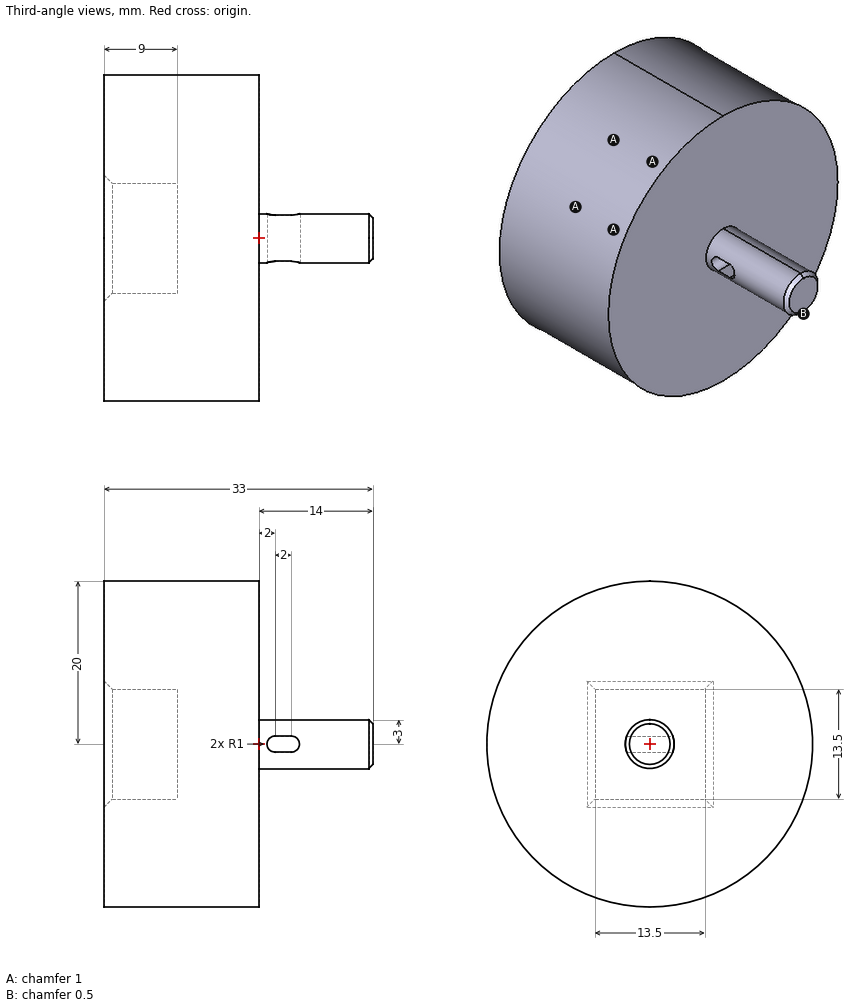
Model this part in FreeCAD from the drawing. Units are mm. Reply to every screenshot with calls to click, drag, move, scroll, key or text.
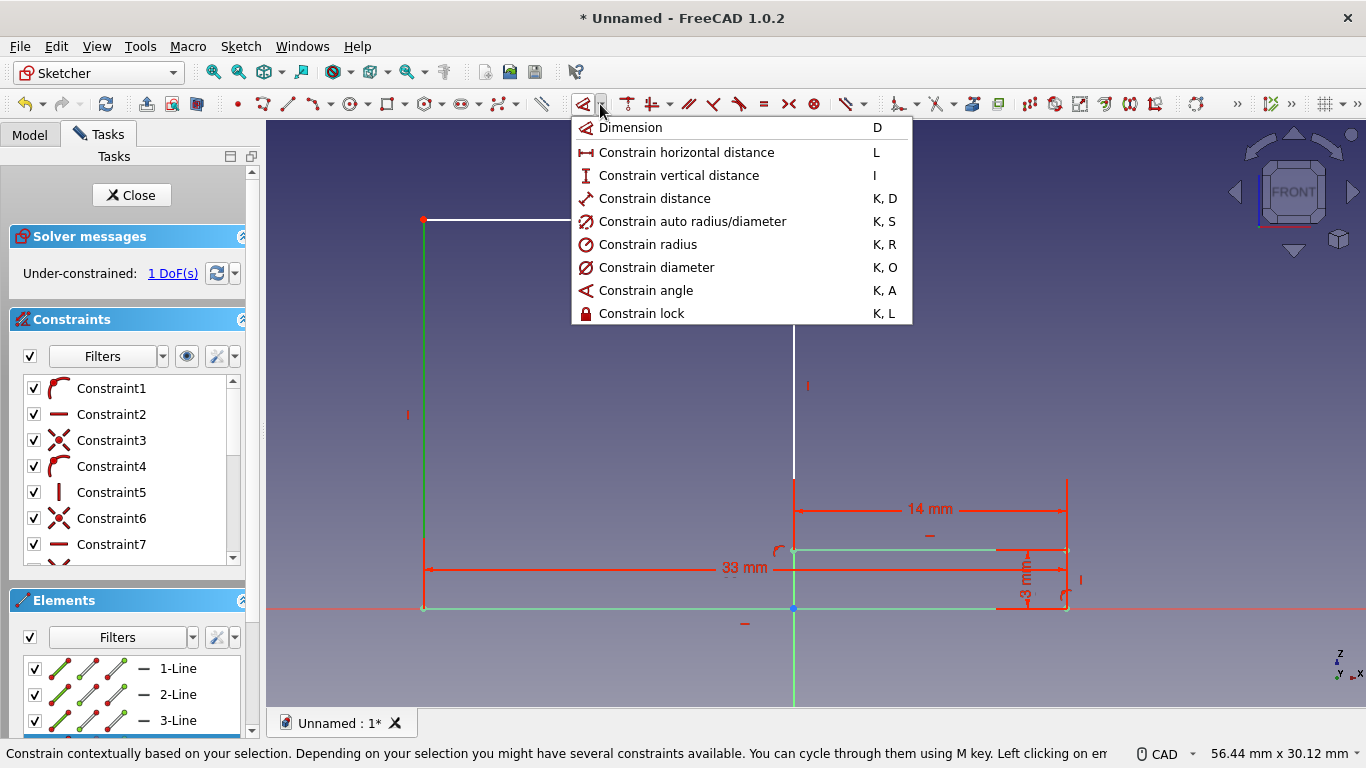
click(742, 176)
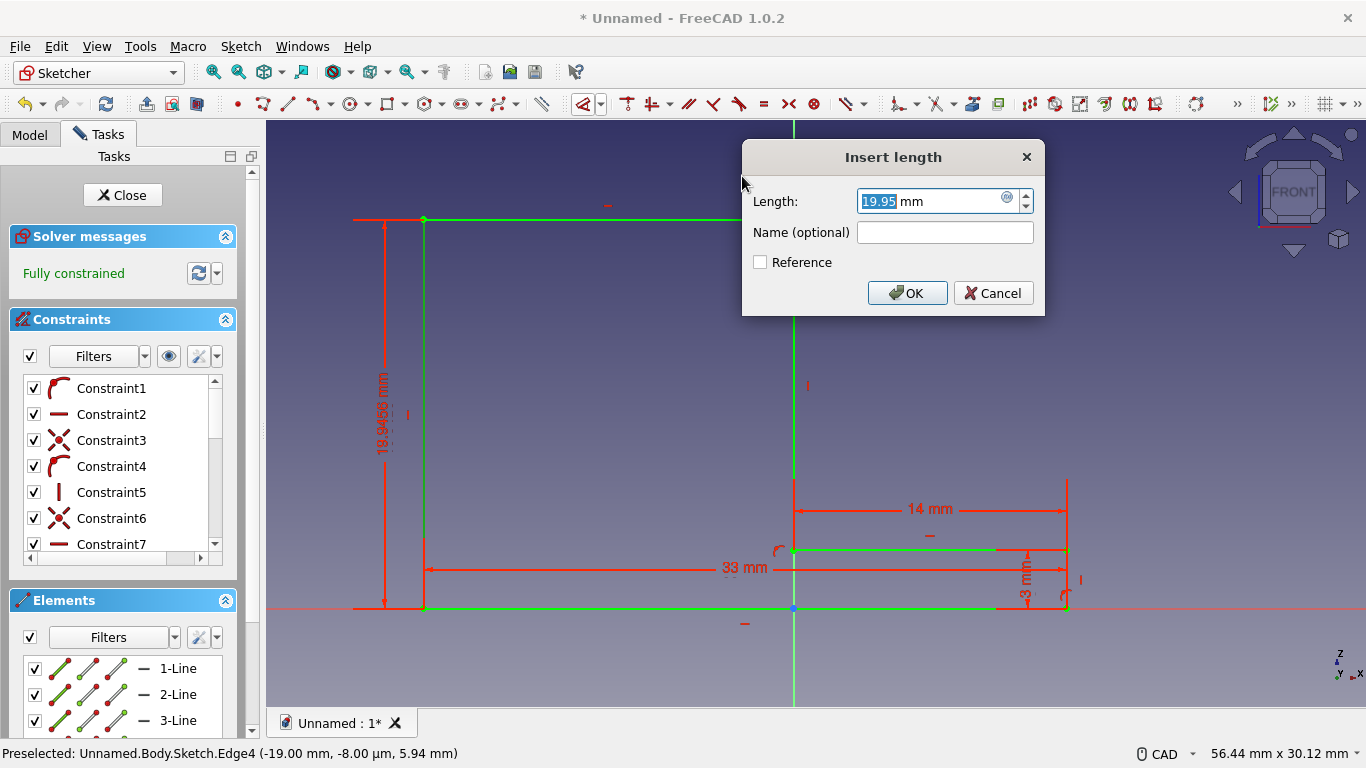
text(20)
key(Return)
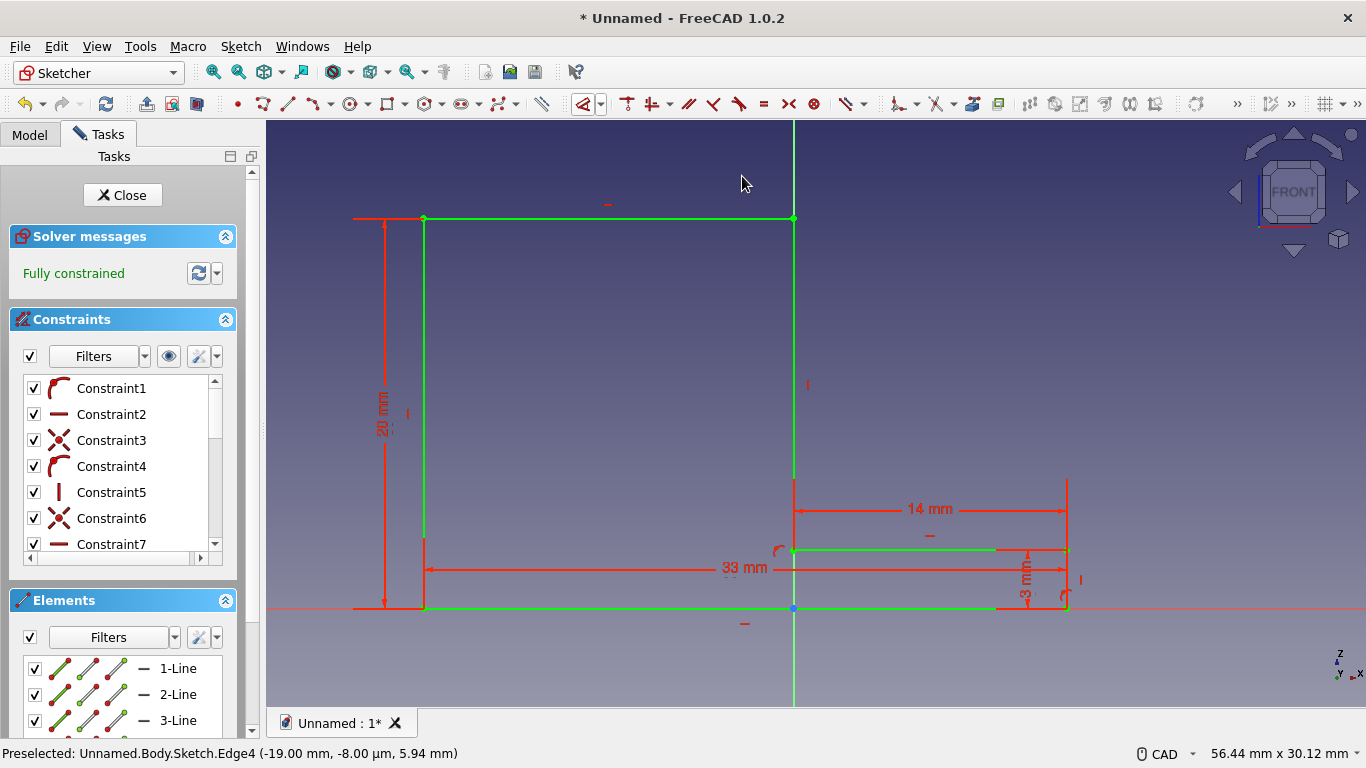
click(123, 195)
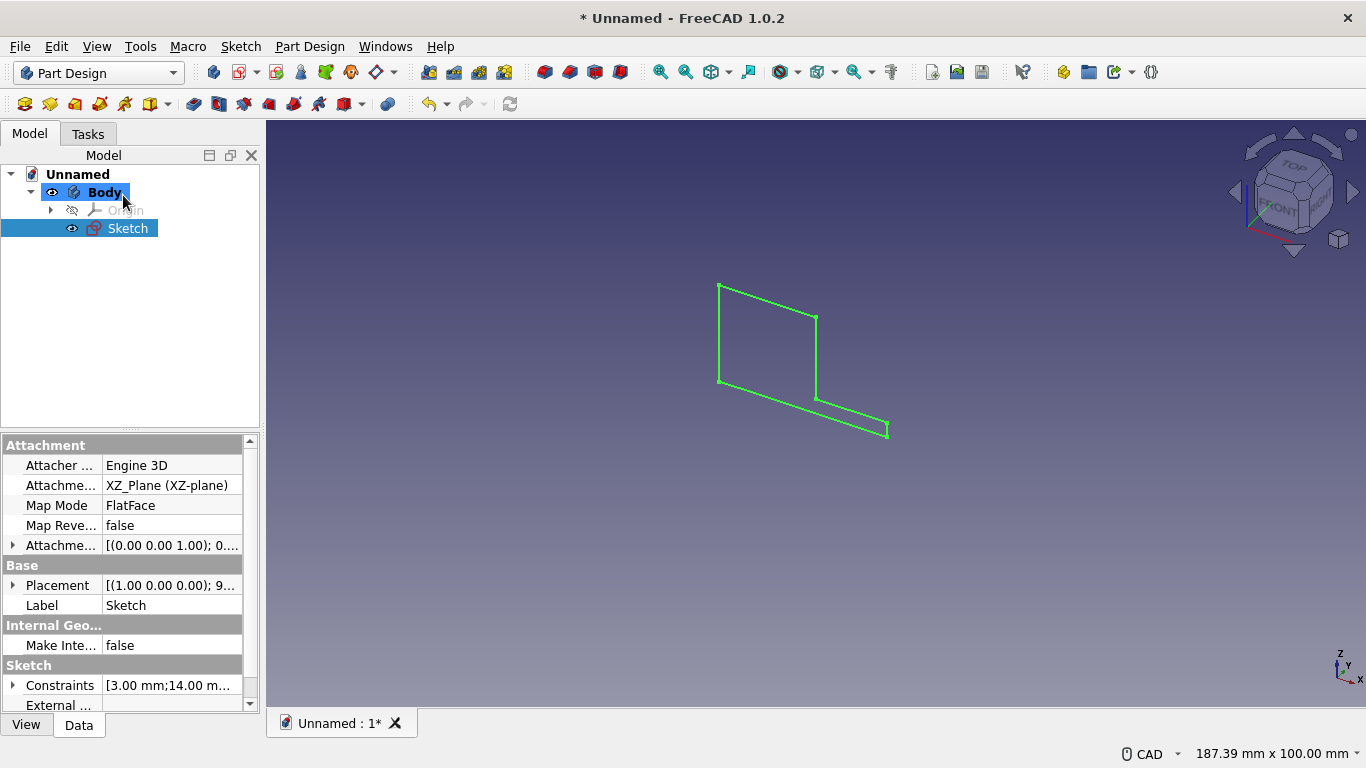
click(50, 104)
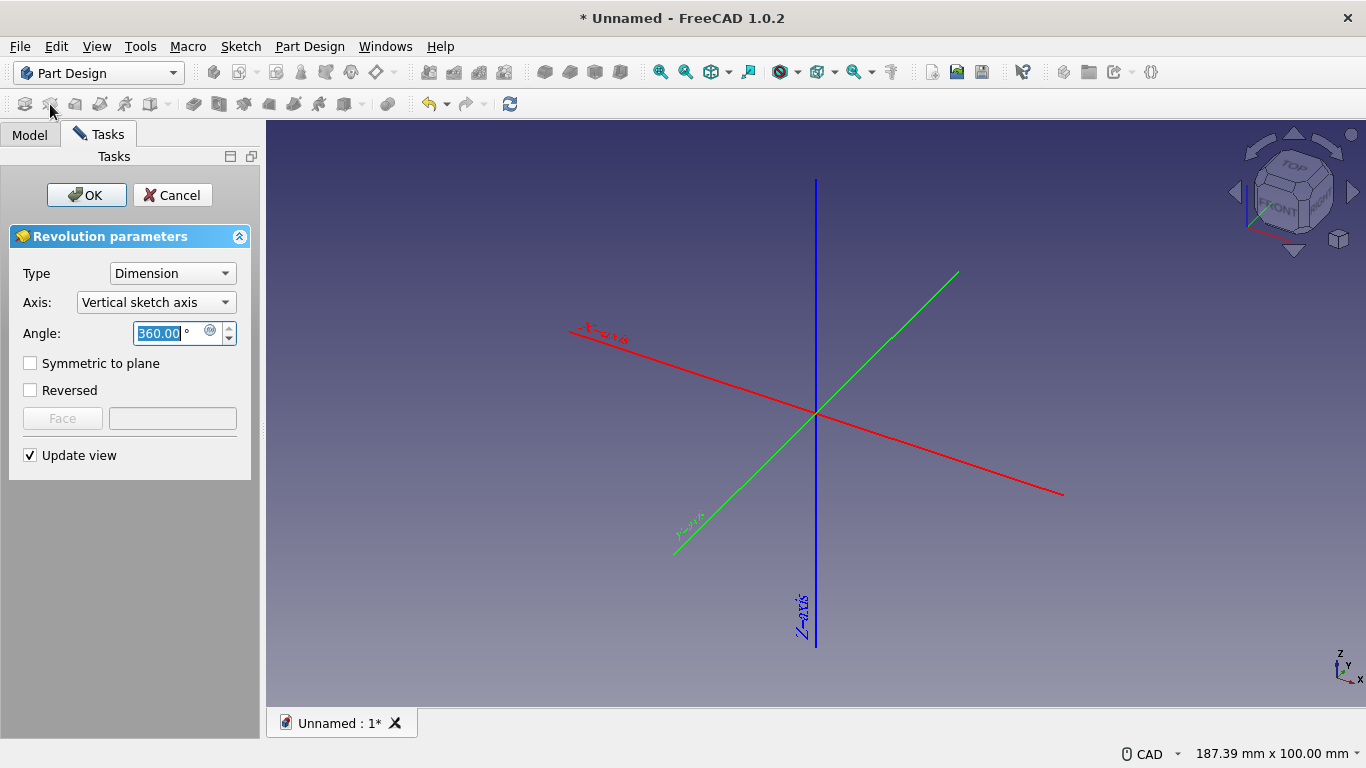
click(157, 302)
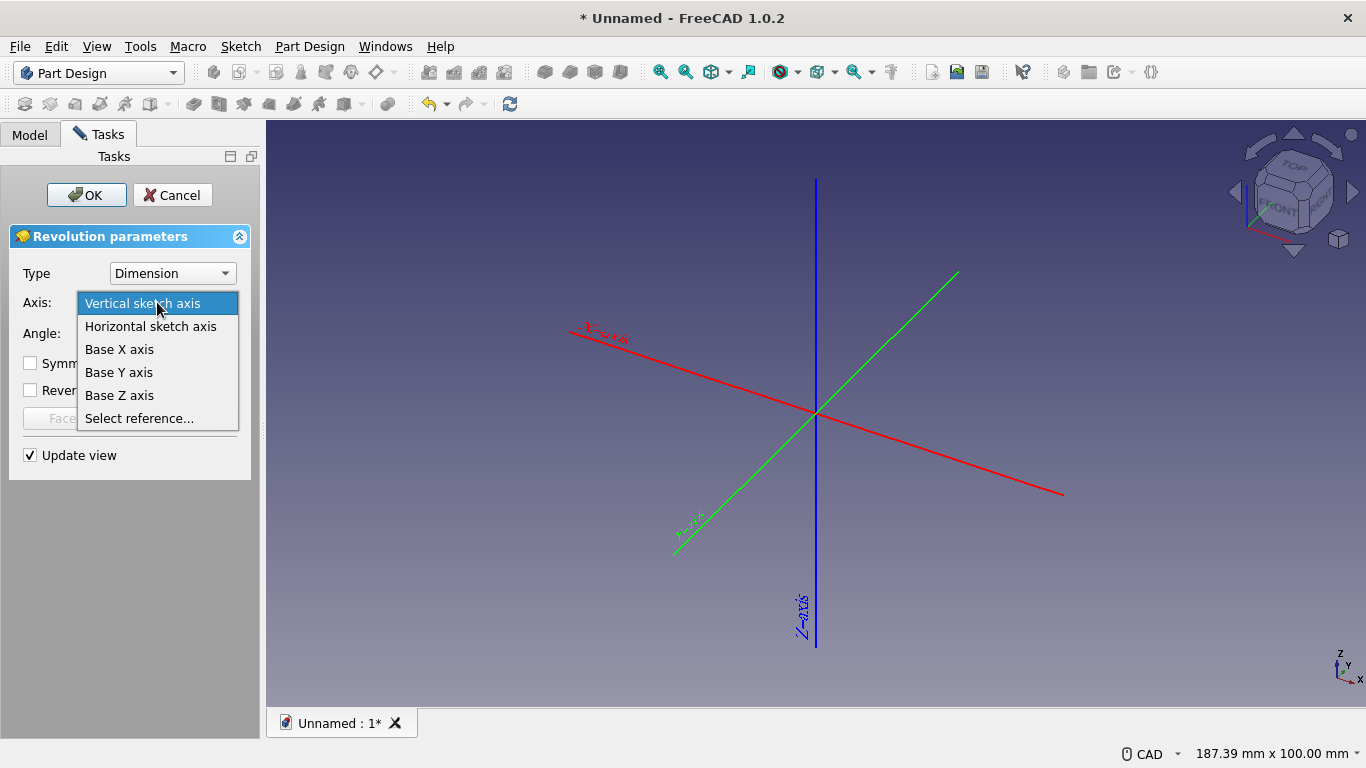
click(156, 326)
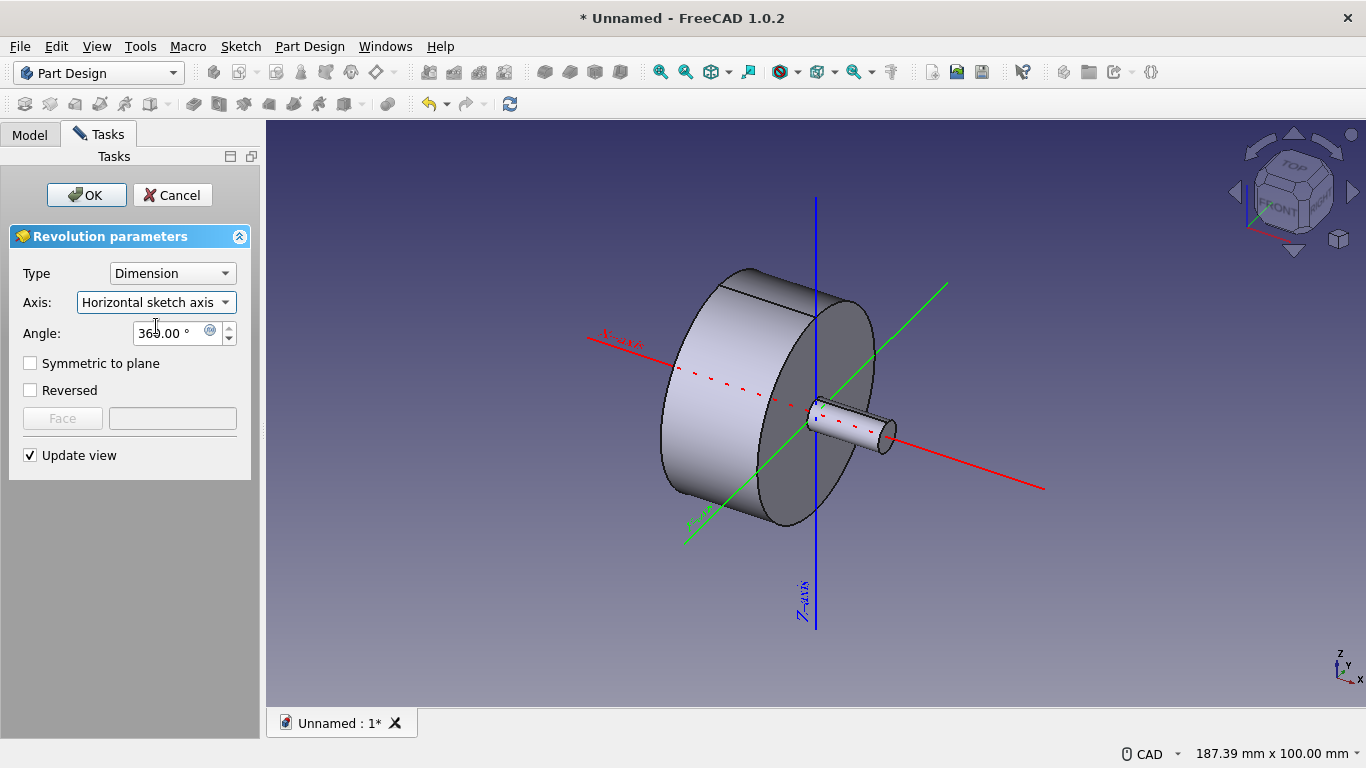
click(87, 195)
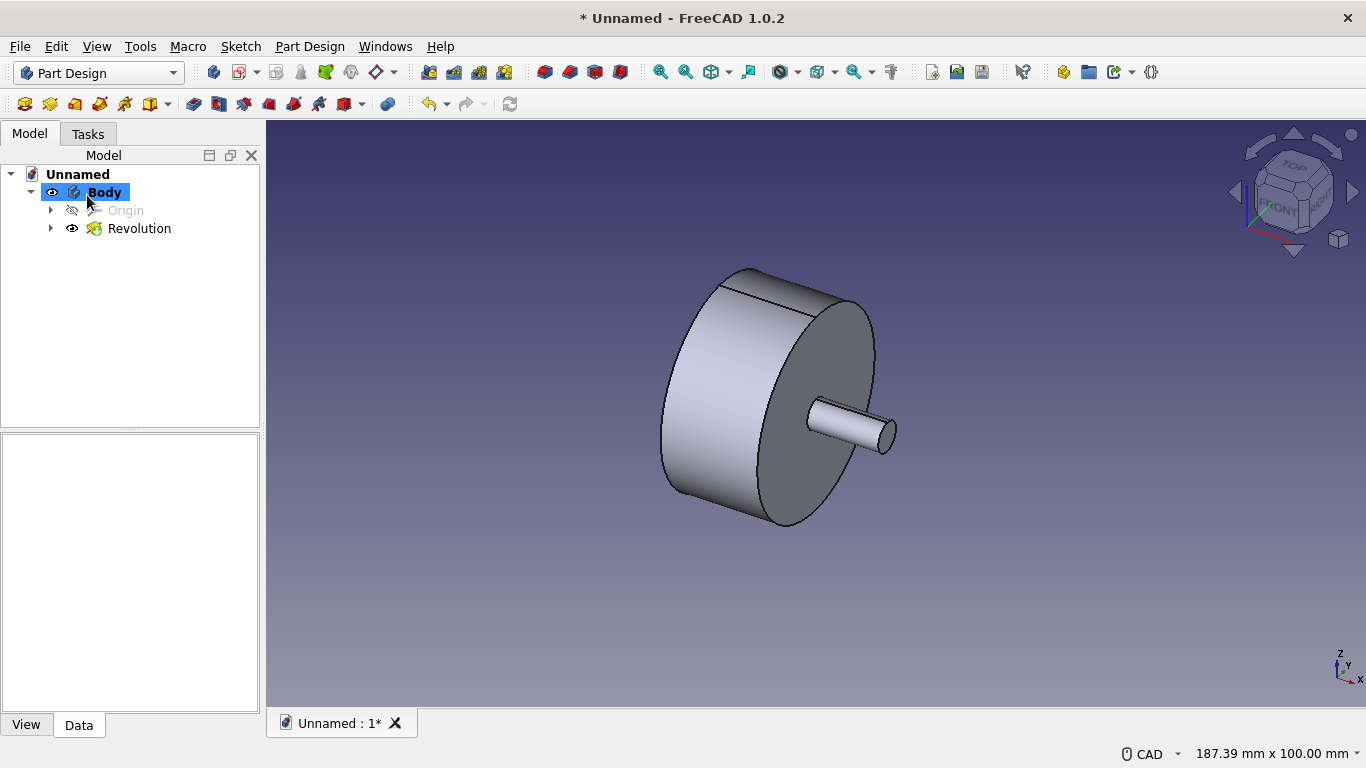
key(6)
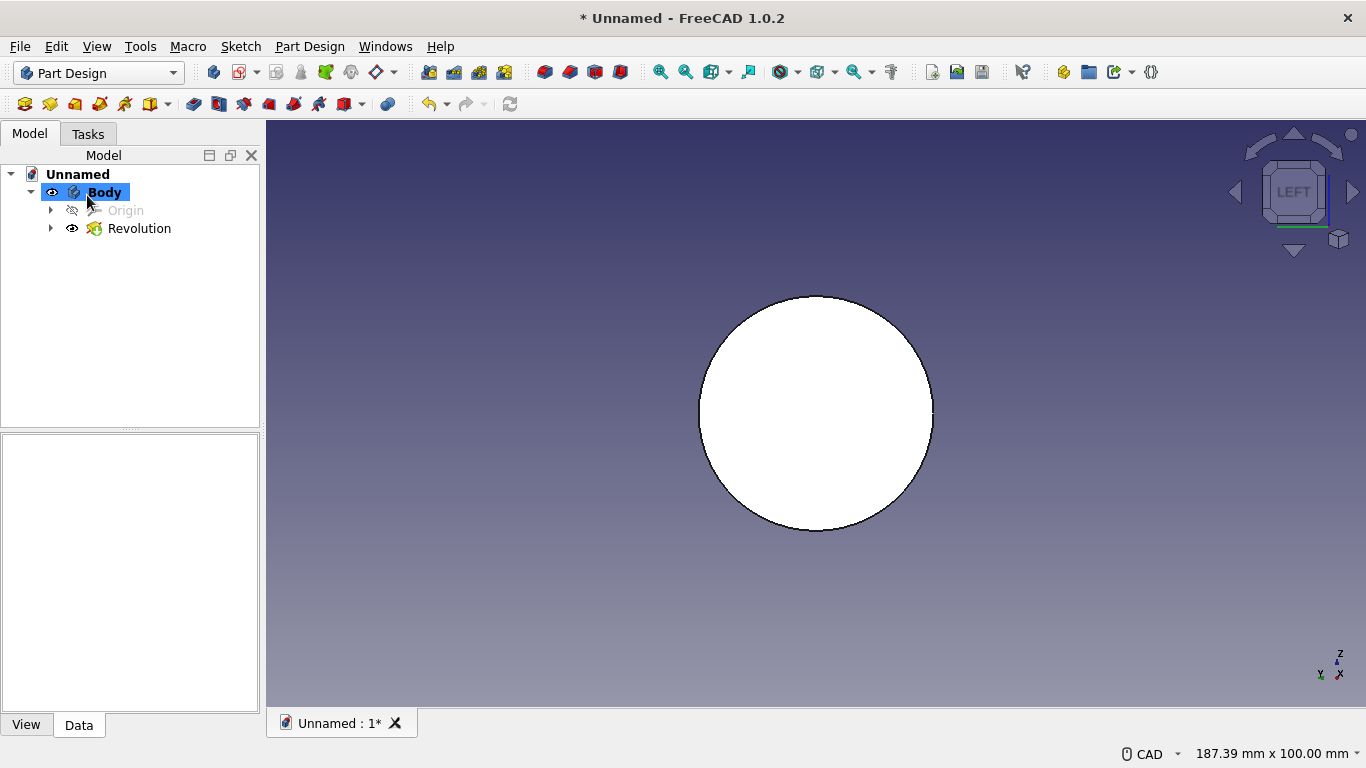
click(661, 72)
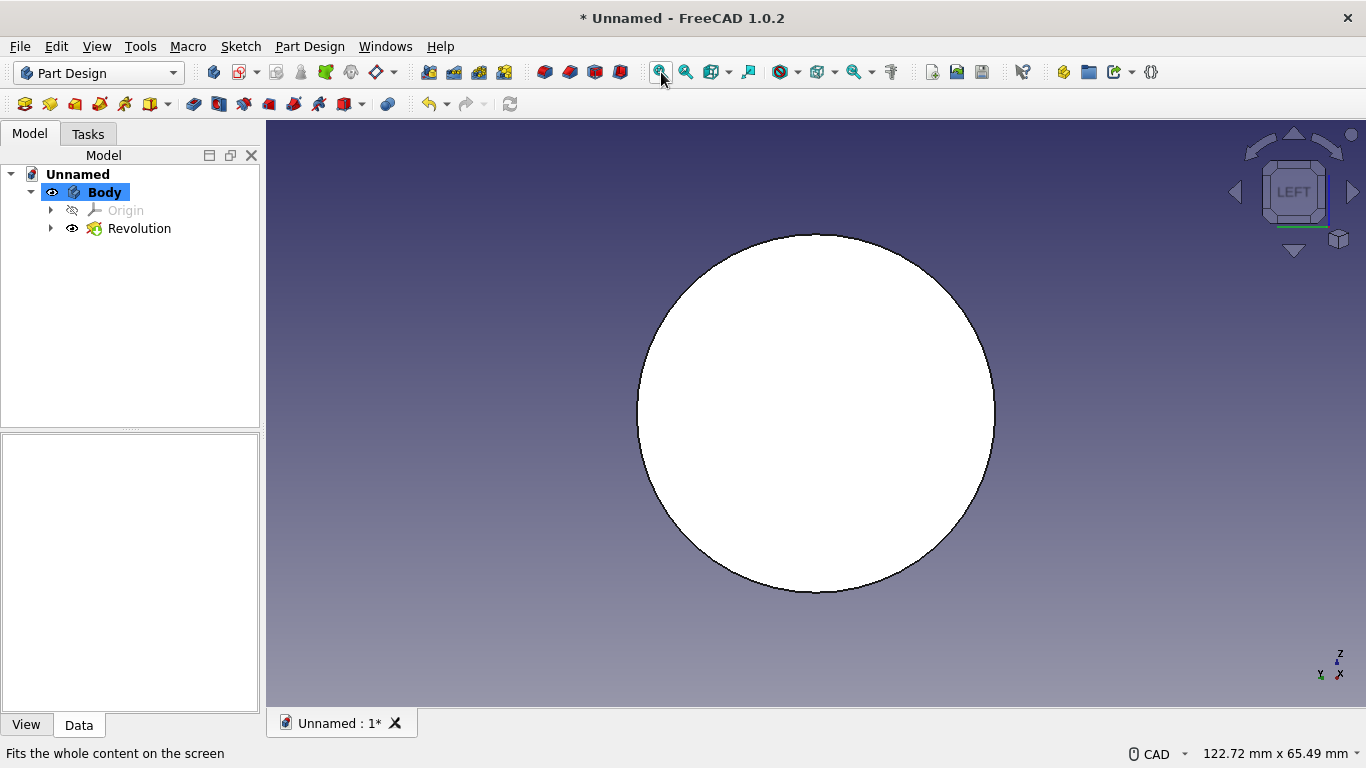
click(816, 412)